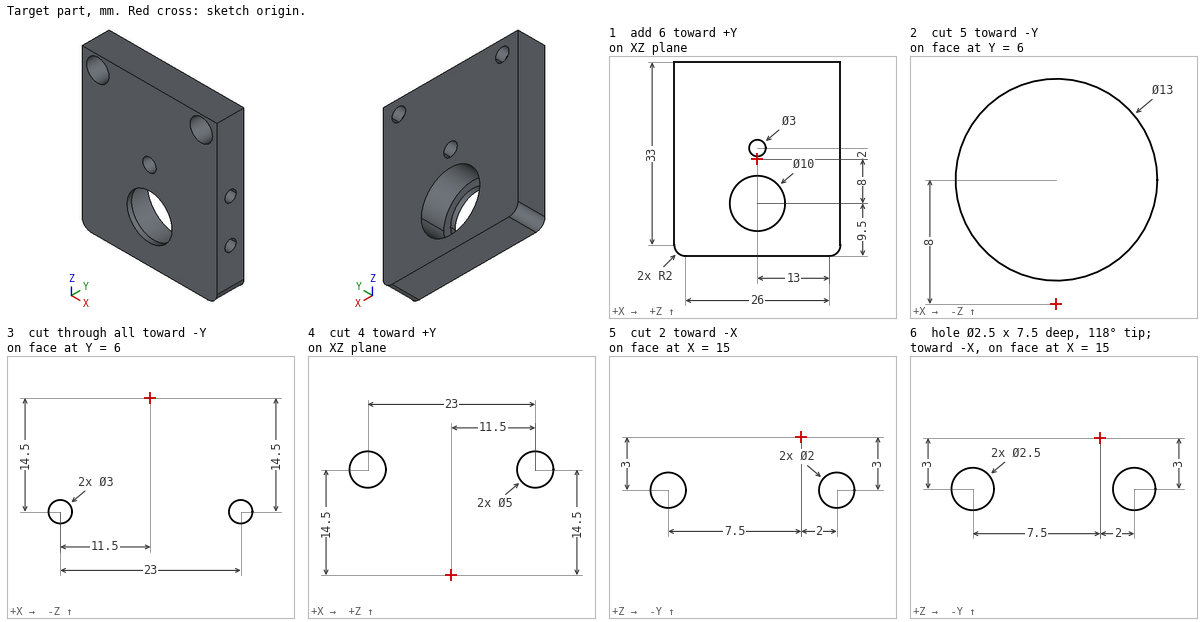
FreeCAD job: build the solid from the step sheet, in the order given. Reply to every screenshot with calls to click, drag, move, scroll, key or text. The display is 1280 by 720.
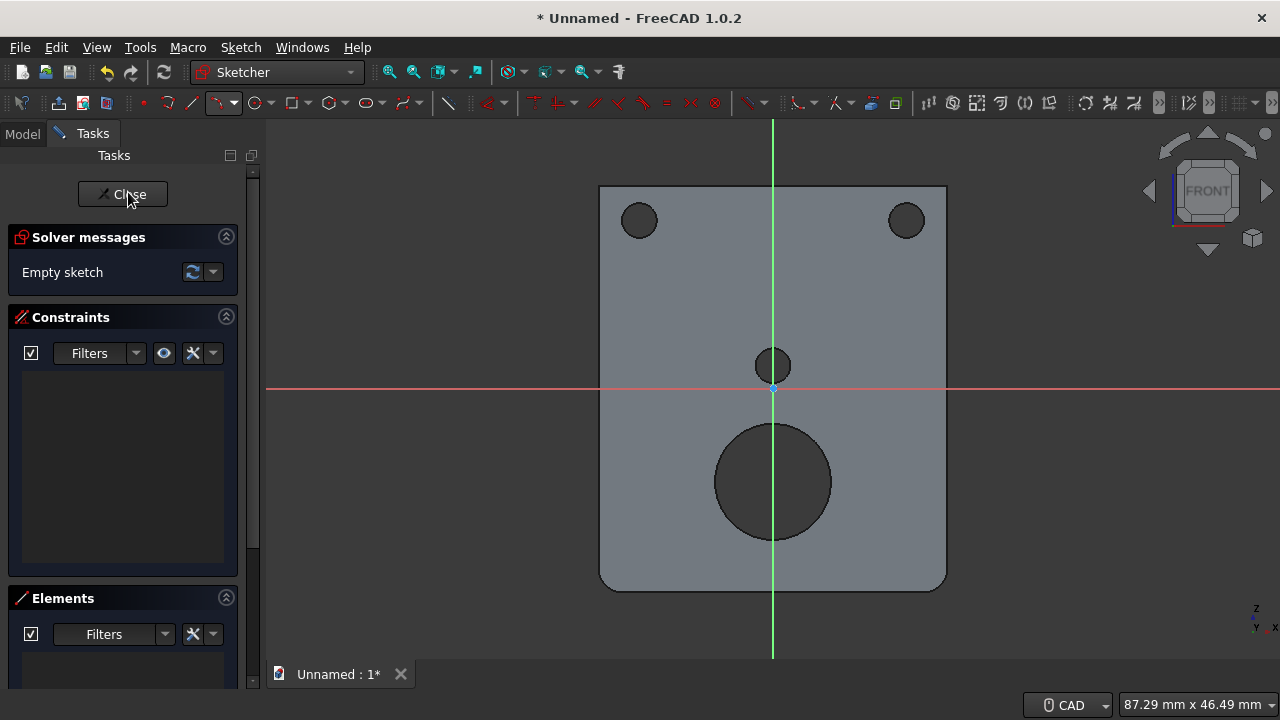
scroll(856, 170, up, 3)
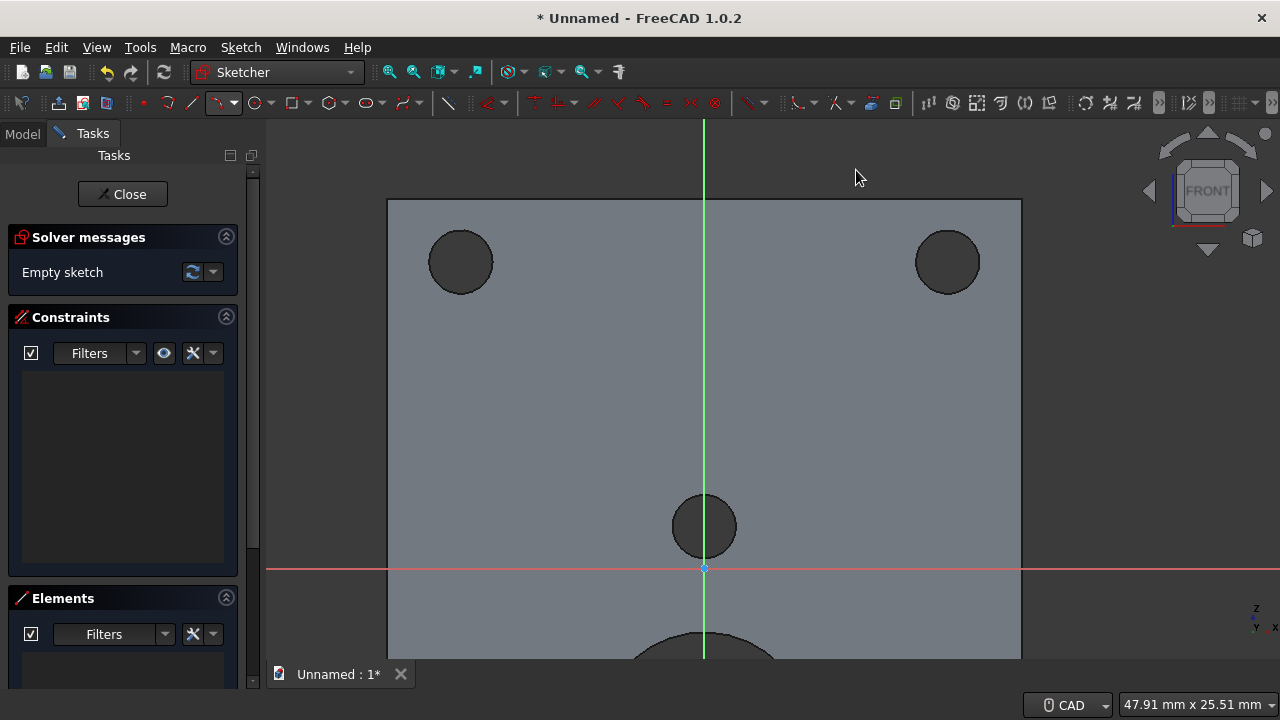
key(g)
key(c)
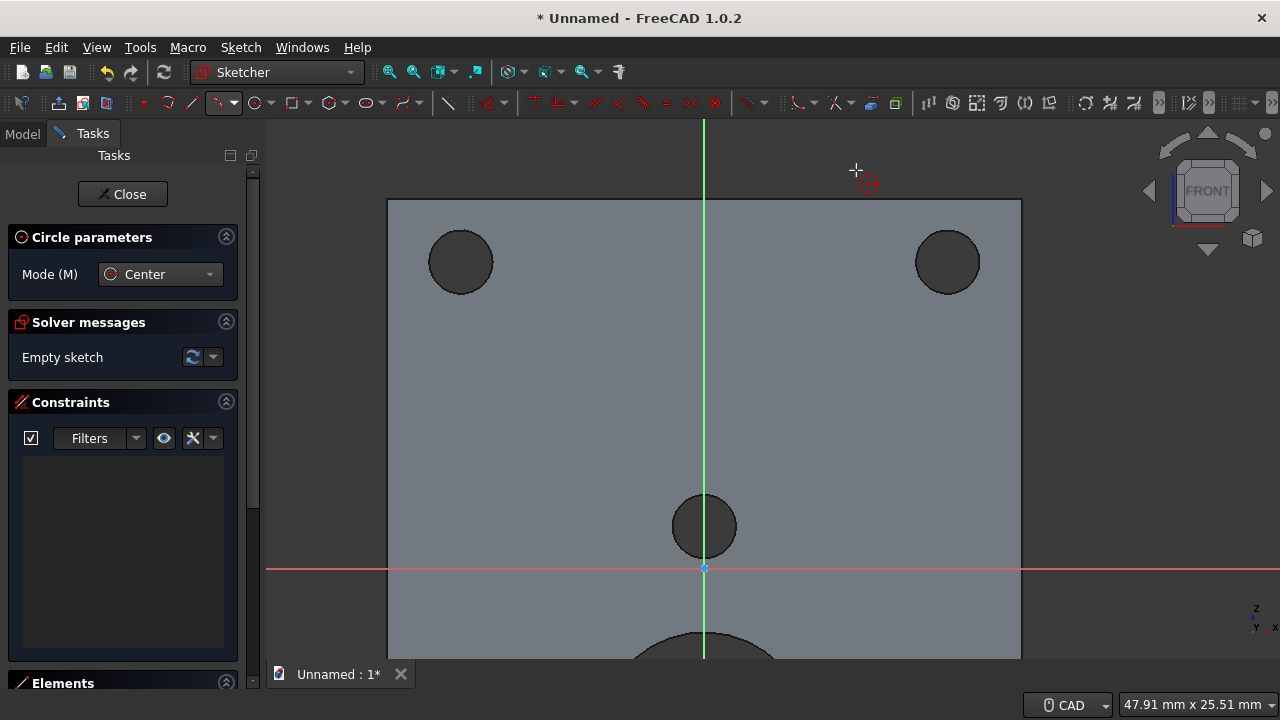
click(948, 262)
click(985, 225)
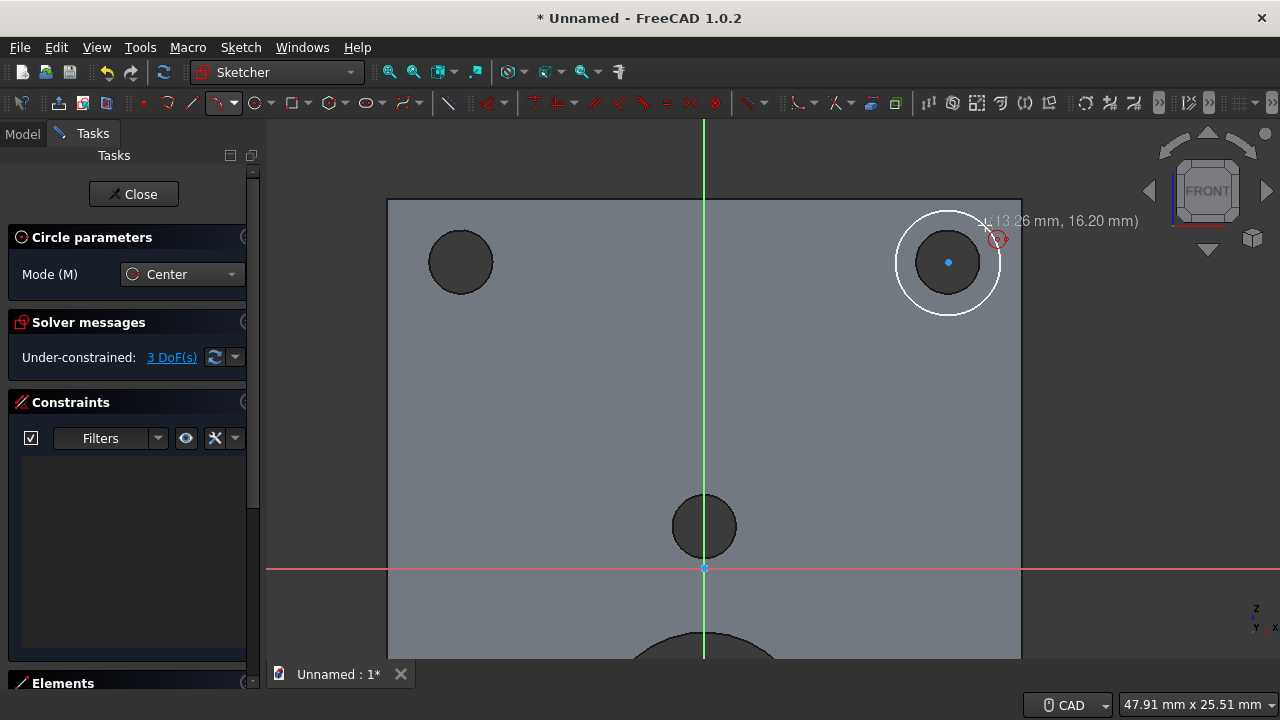
click(461, 262)
click(498, 225)
key(Escape)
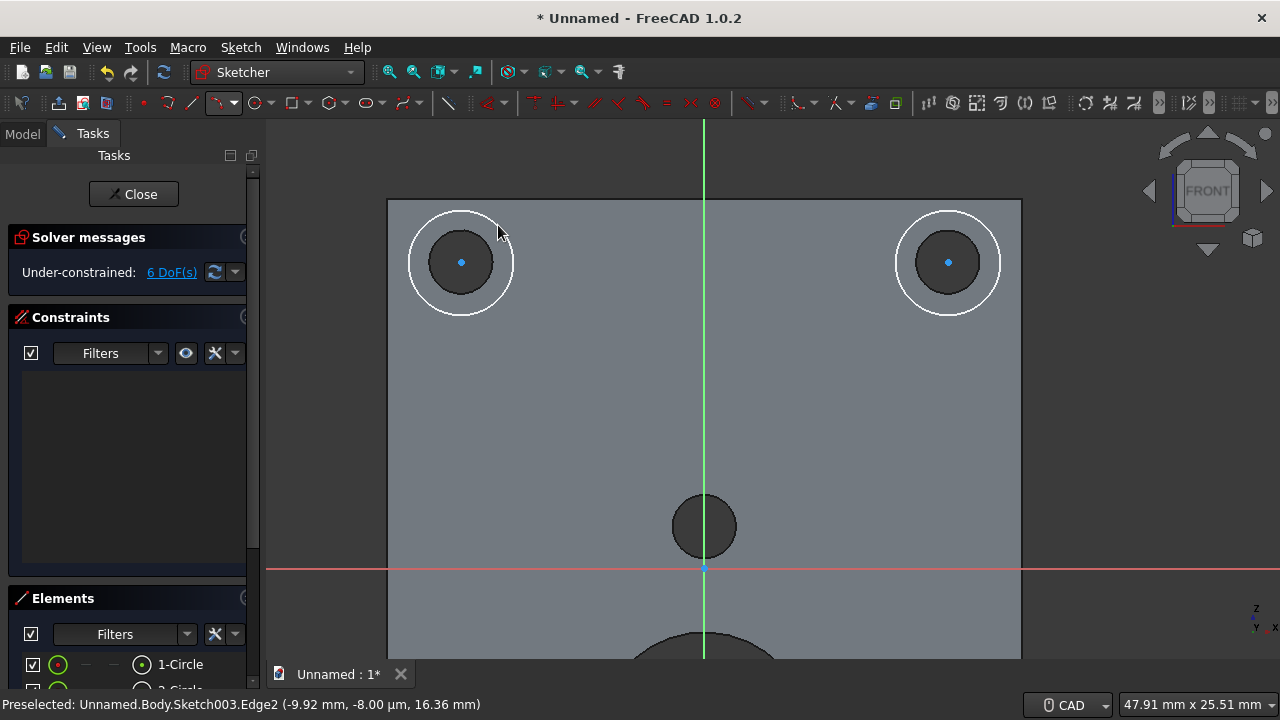
click(985, 226)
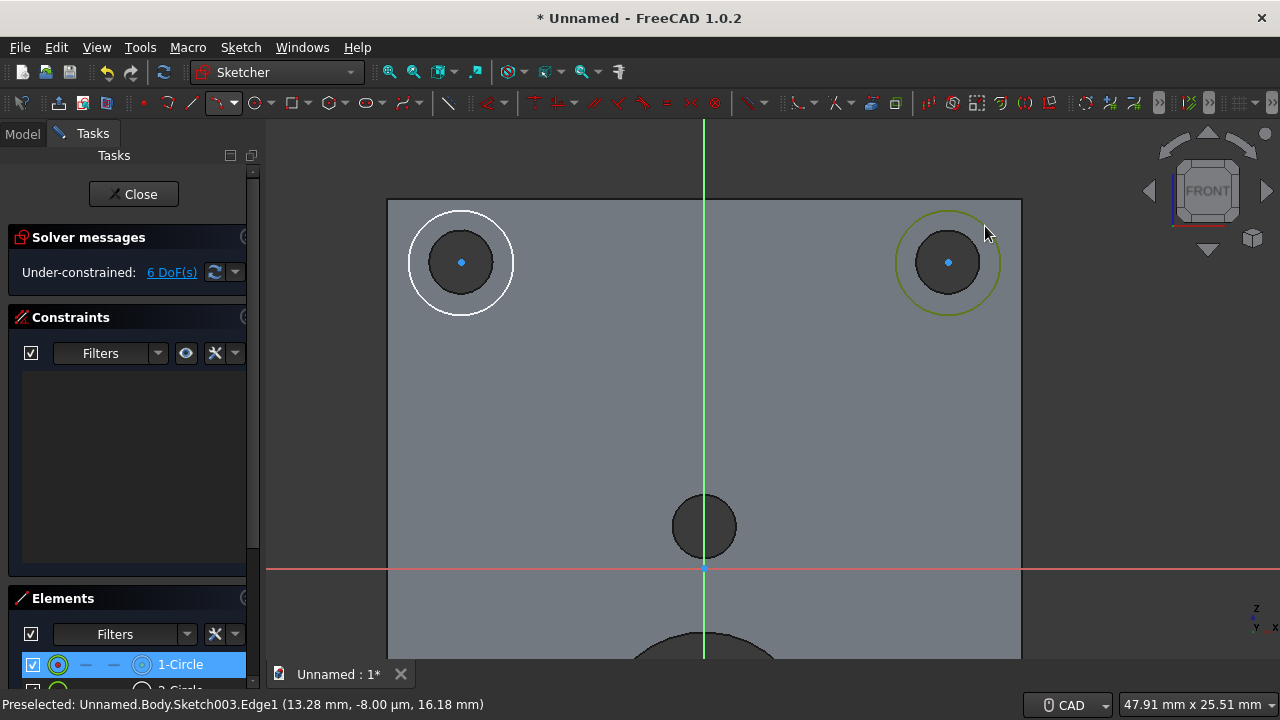
click(498, 226)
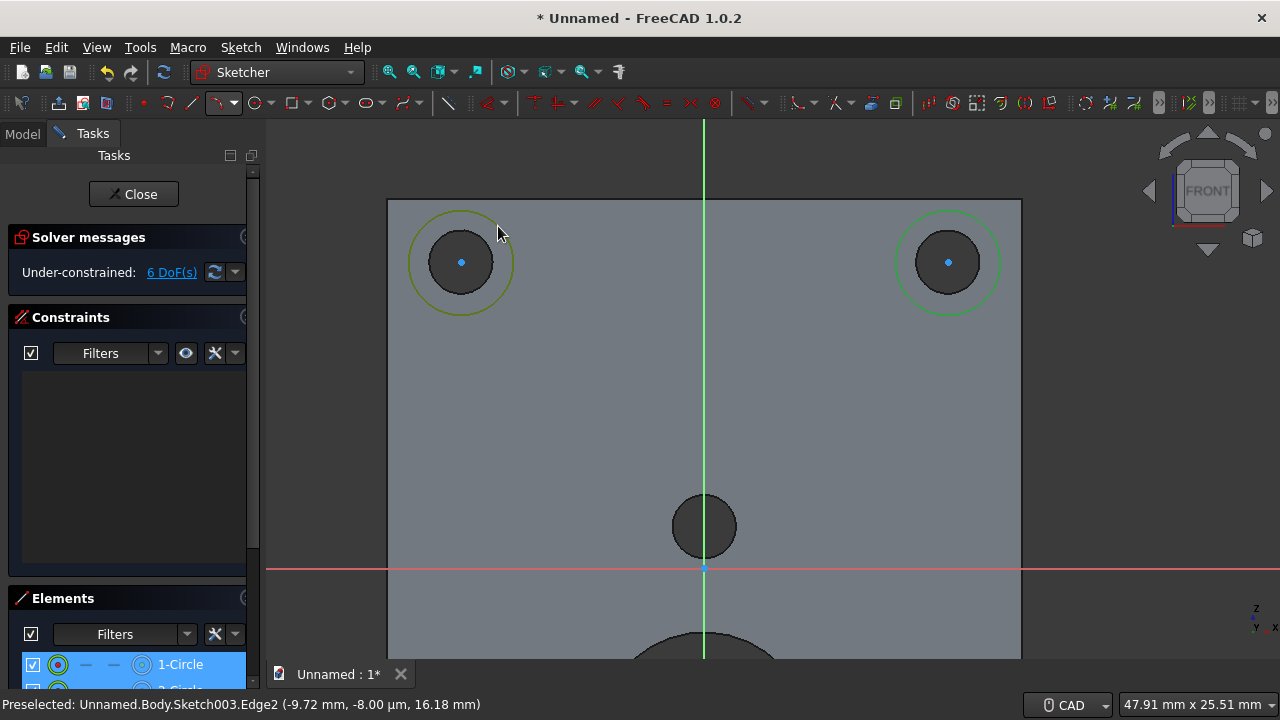
click(668, 104)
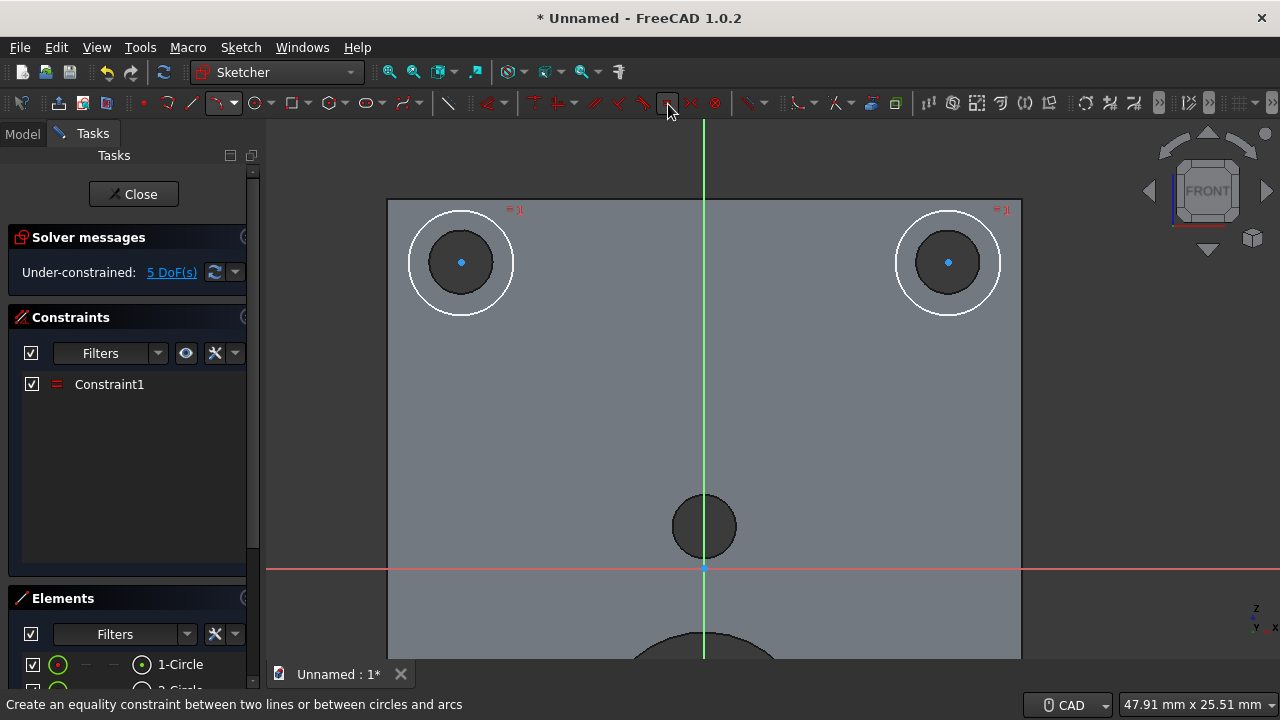
key(d)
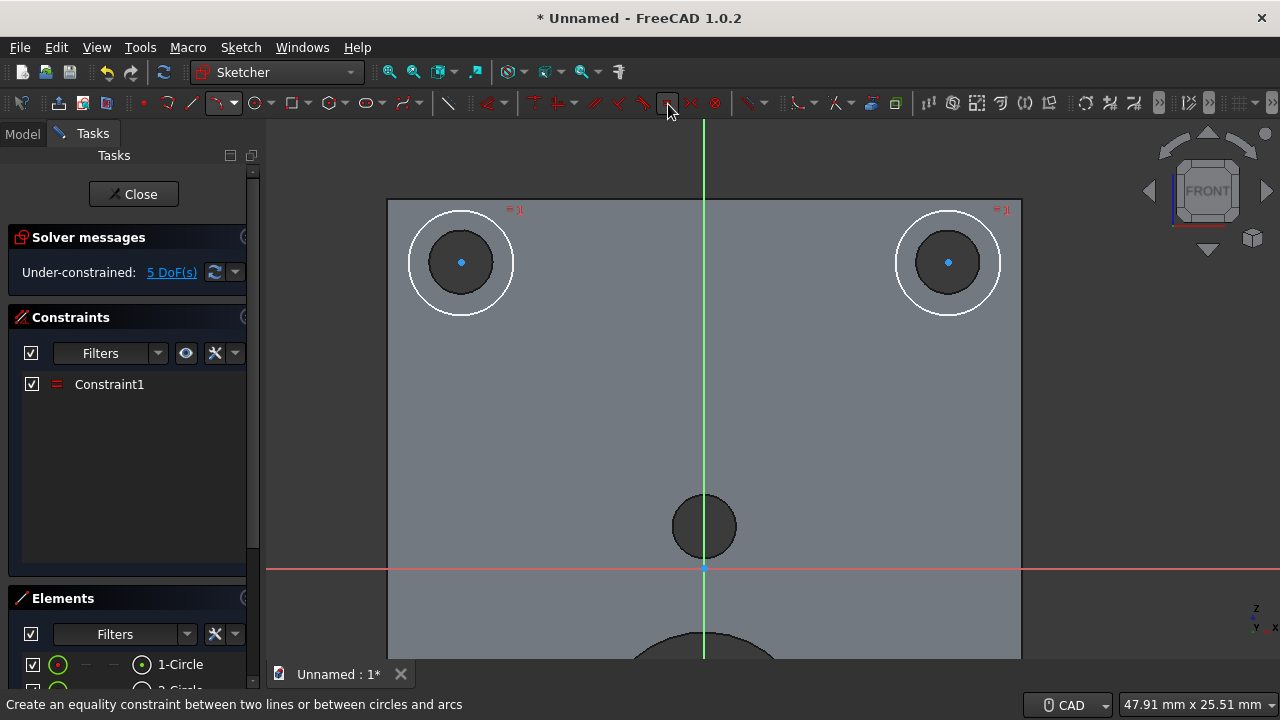
click(985, 226)
click(1008, 203)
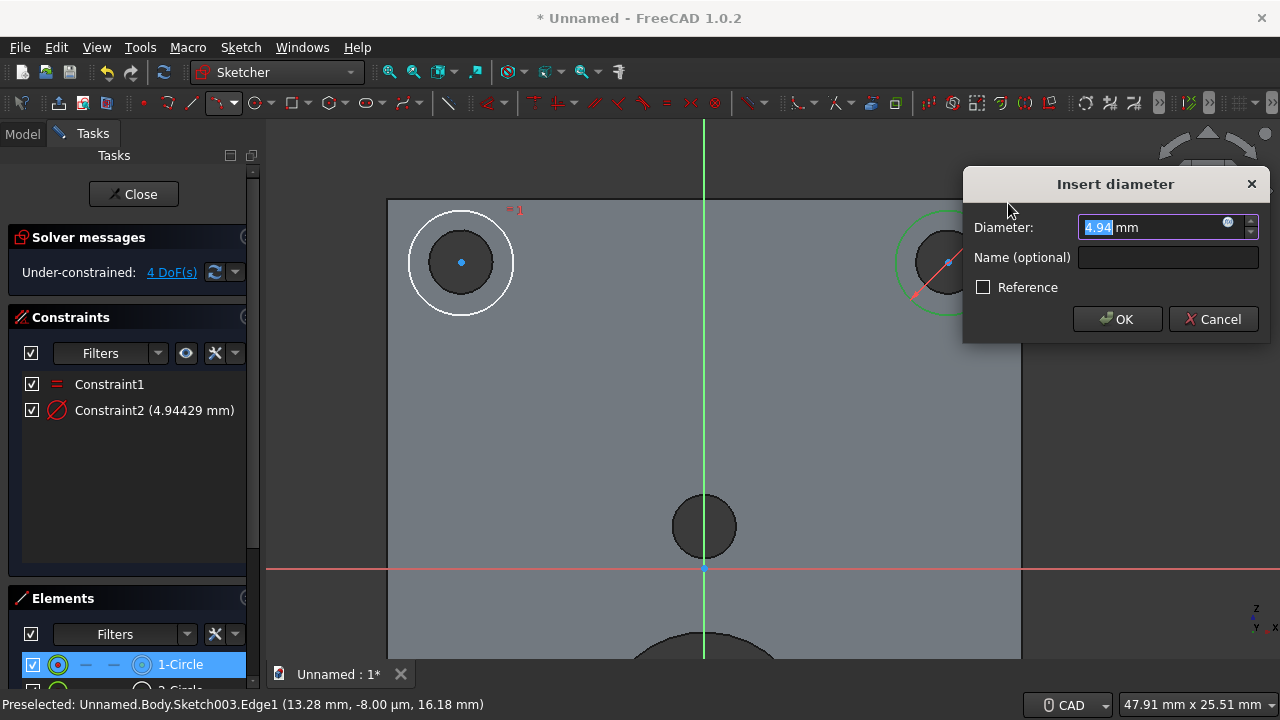
text(5)
key(Return)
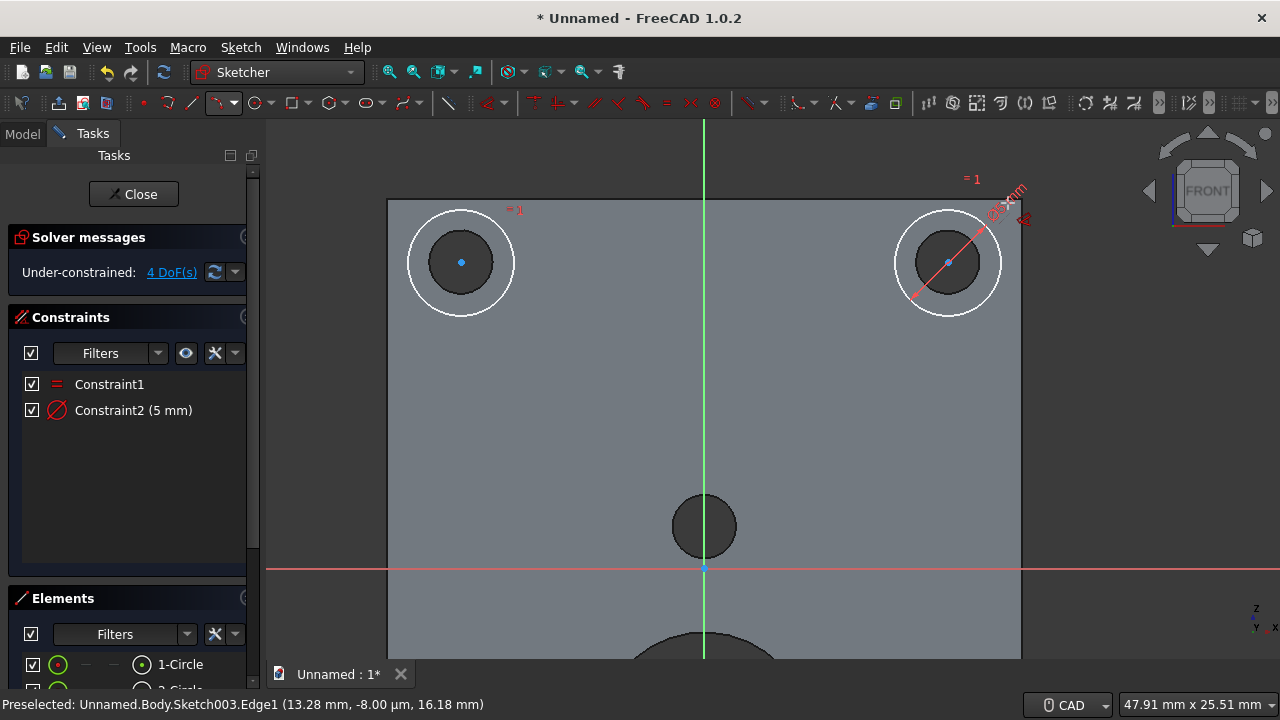
click(948, 263)